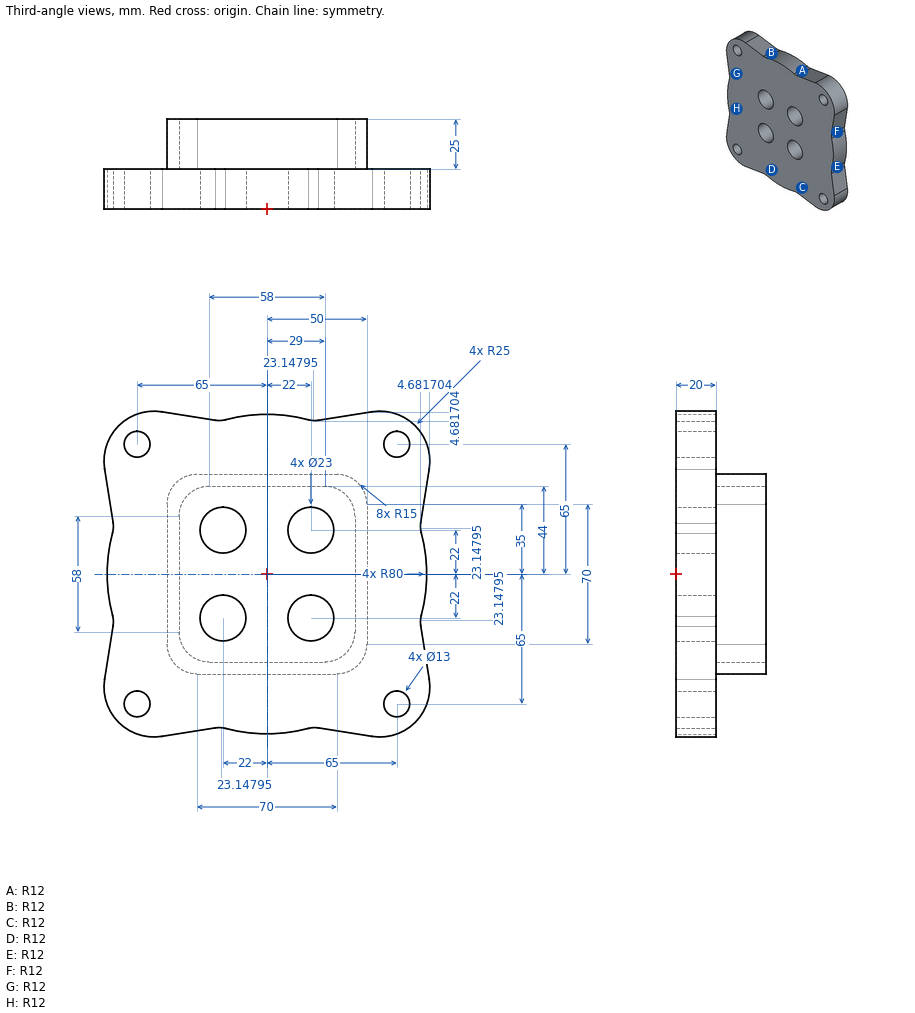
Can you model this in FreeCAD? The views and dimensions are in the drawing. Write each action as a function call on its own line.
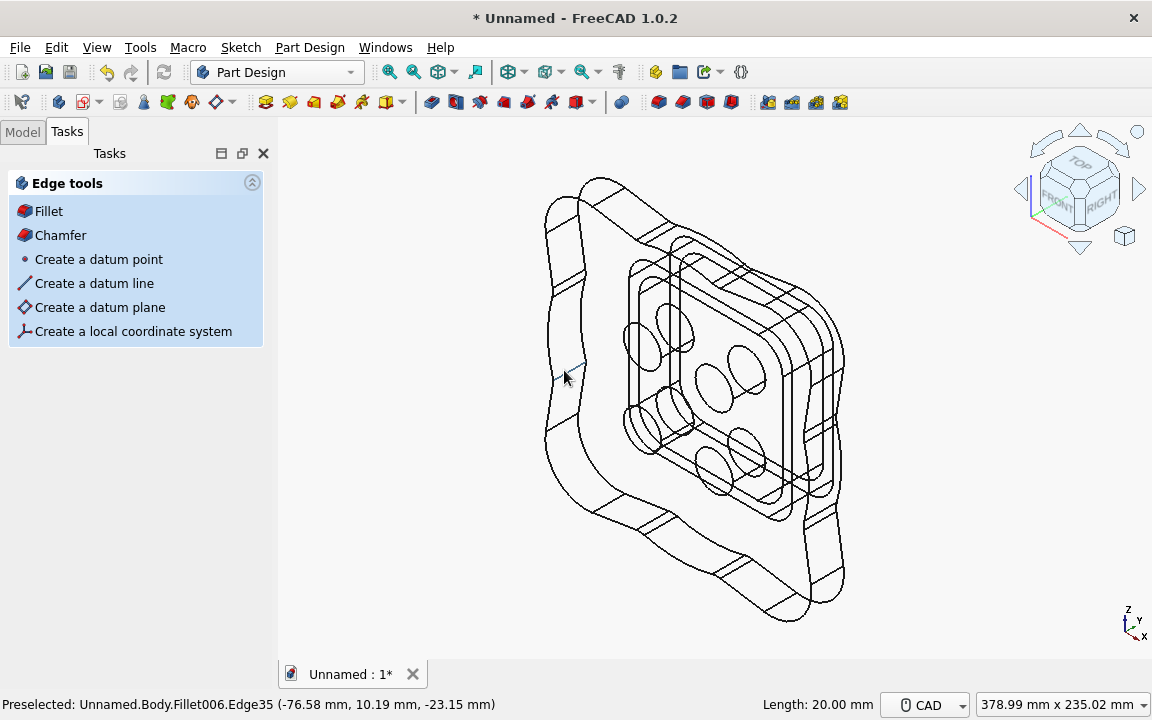
key(v)
key(1)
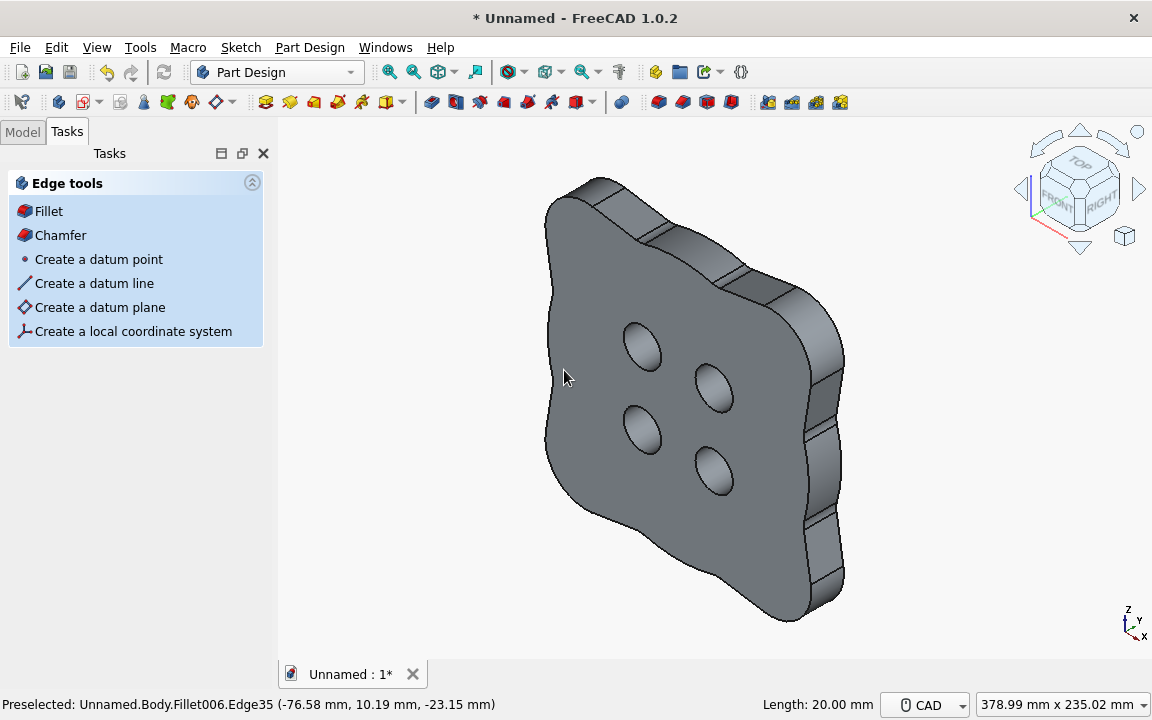
click(660, 102)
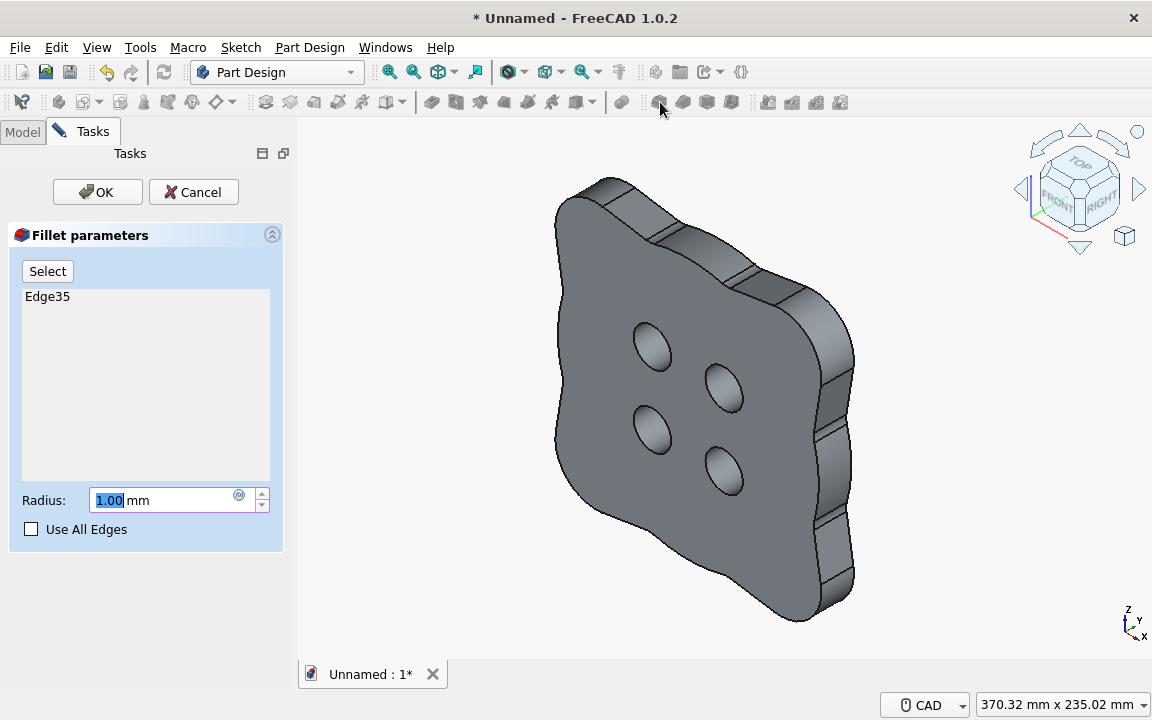
text(12)
key(Tab)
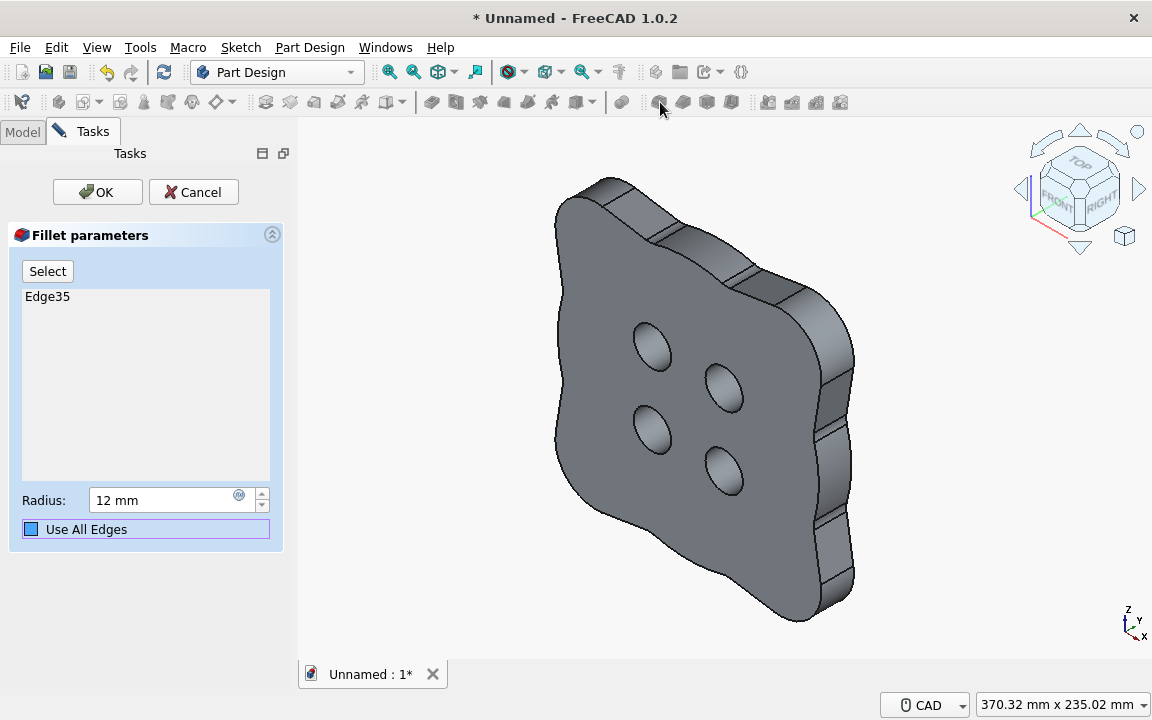
click(98, 192)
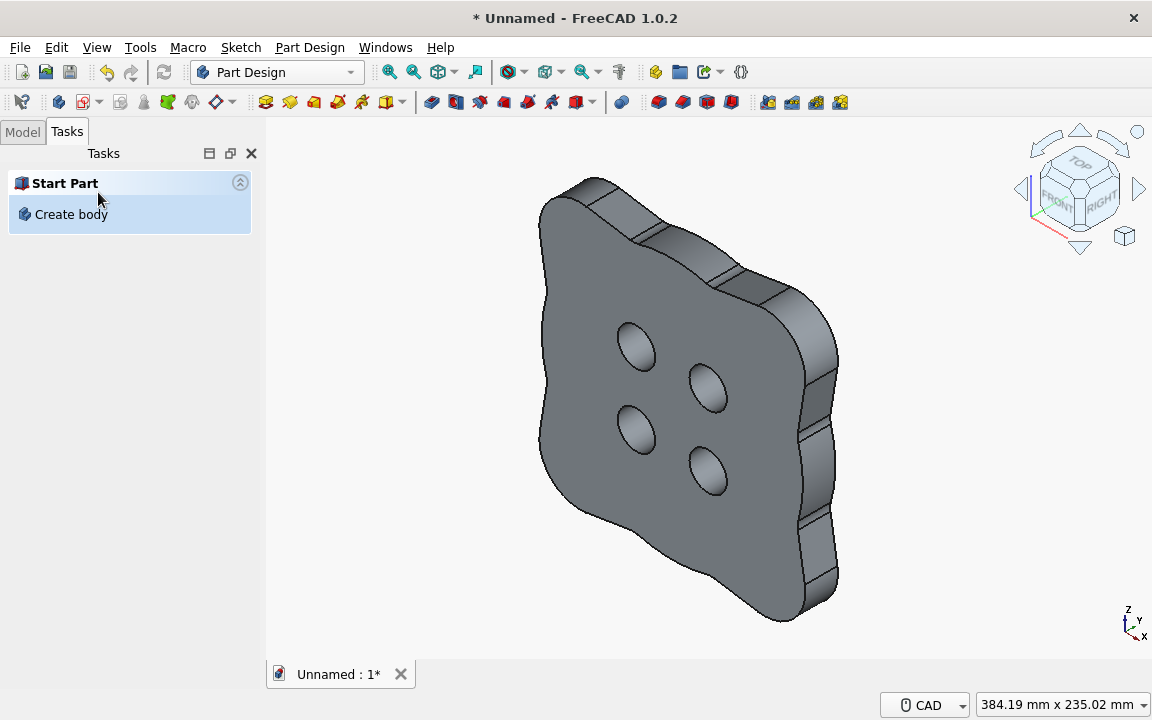
key(4)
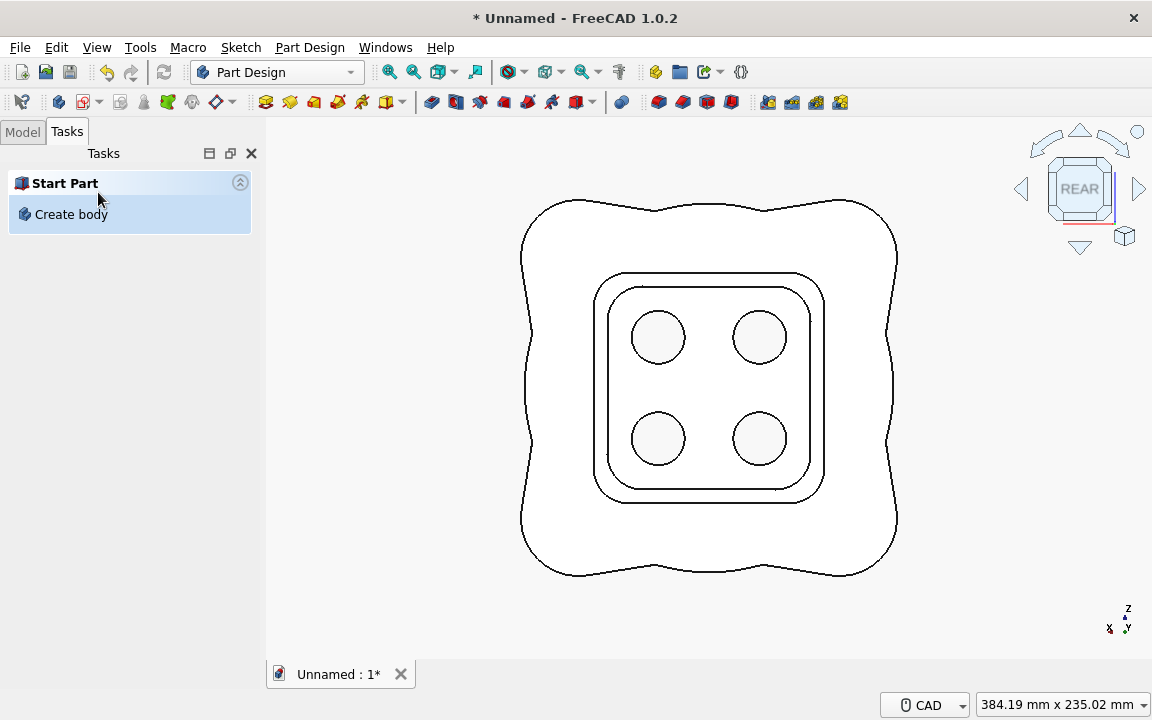
click(816, 548)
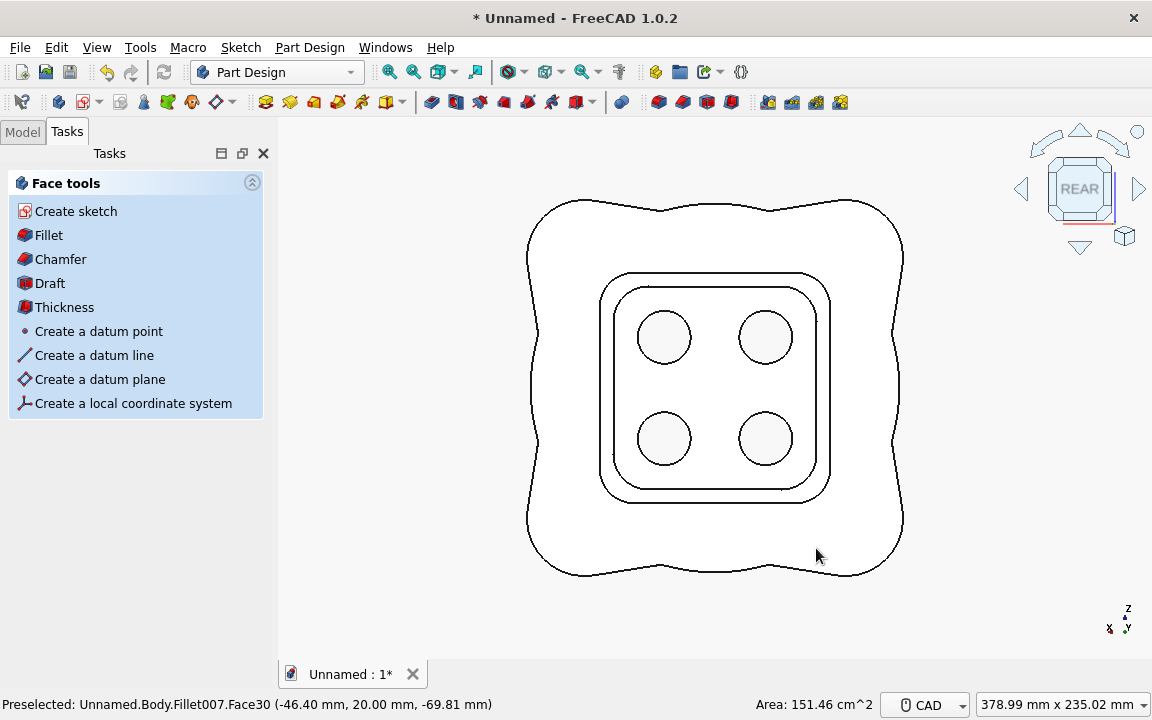
click(84, 102)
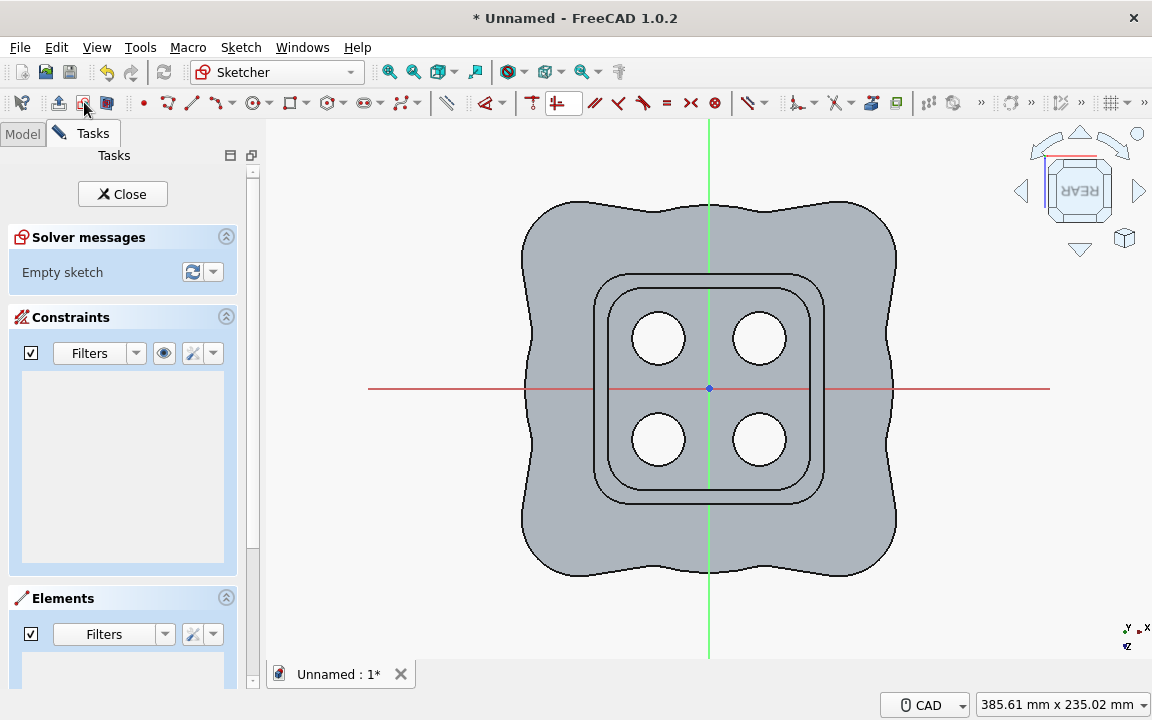
click(254, 104)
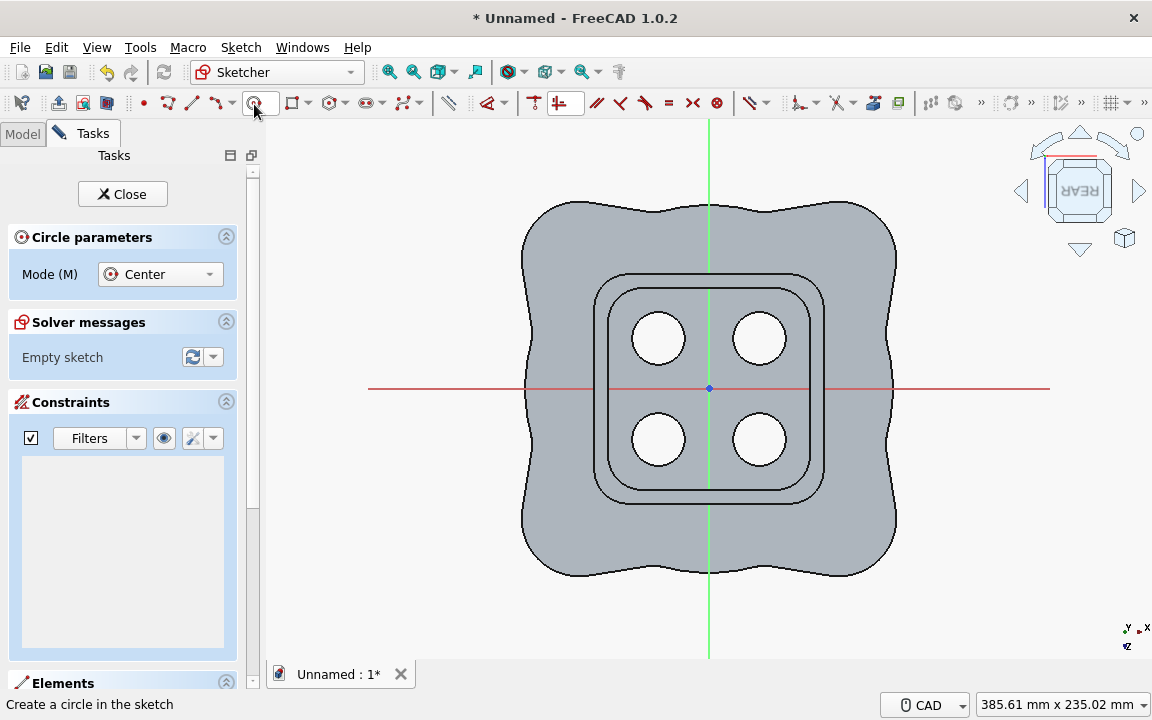
scroll(858, 240, up, 3)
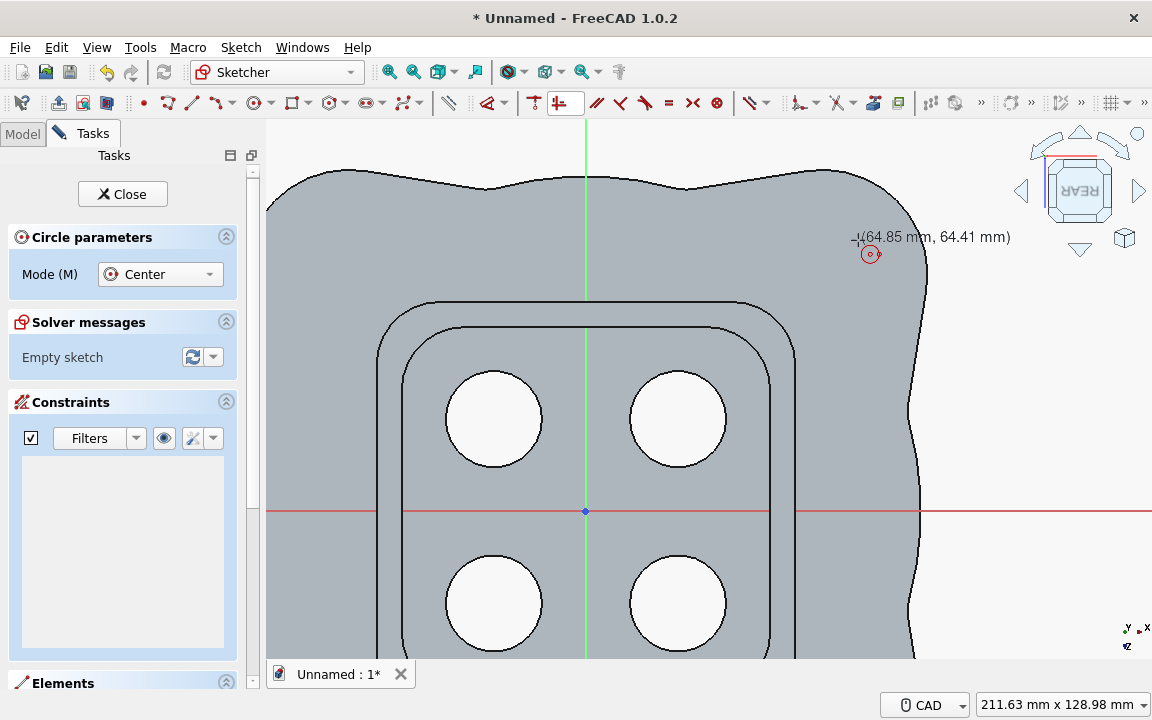
click(858, 239)
move(877, 220)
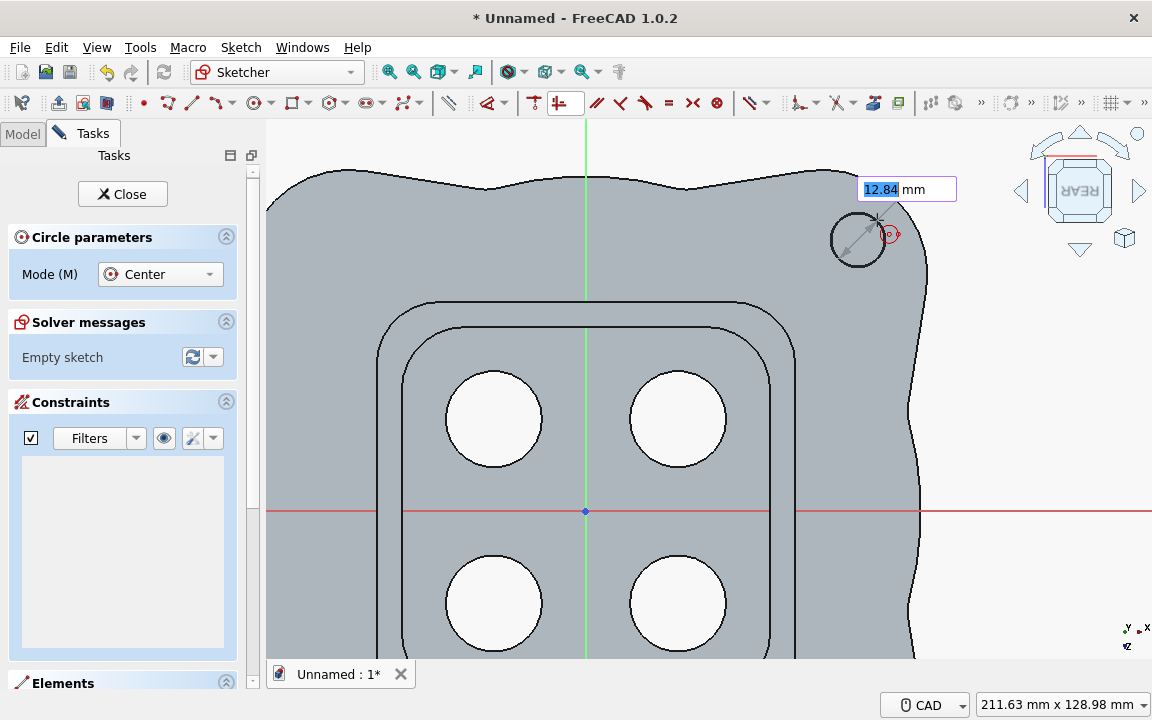
text(13)
key(Return)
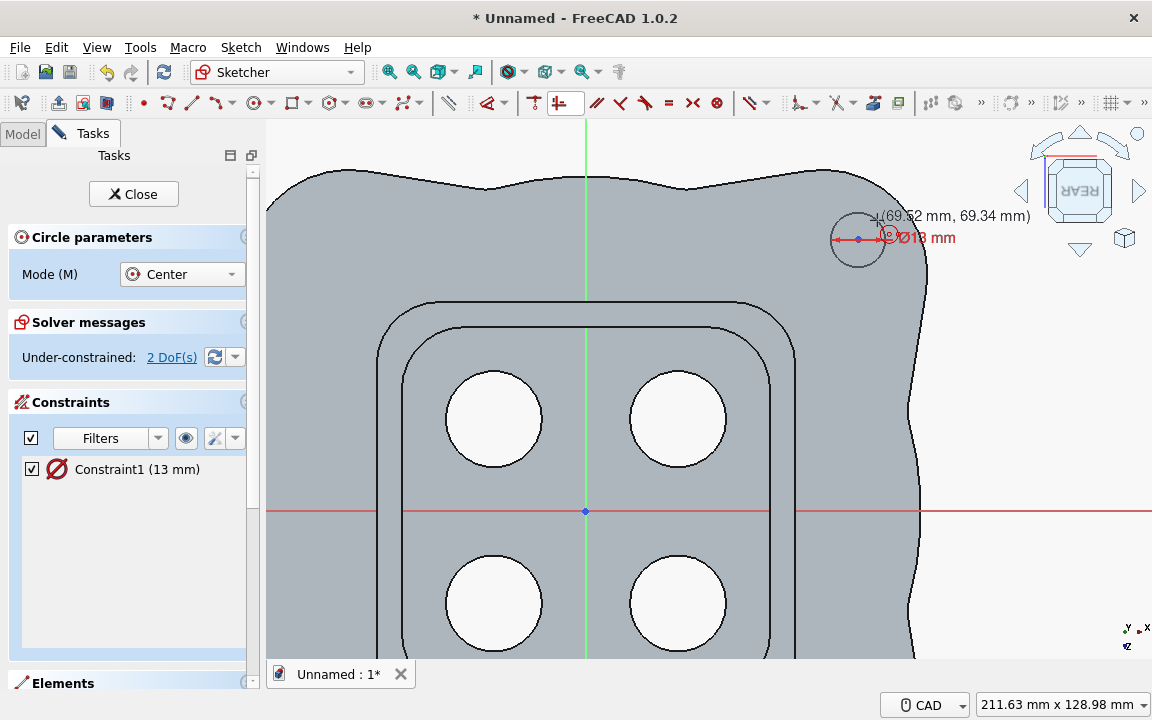
scroll(707, 240, down, 3)